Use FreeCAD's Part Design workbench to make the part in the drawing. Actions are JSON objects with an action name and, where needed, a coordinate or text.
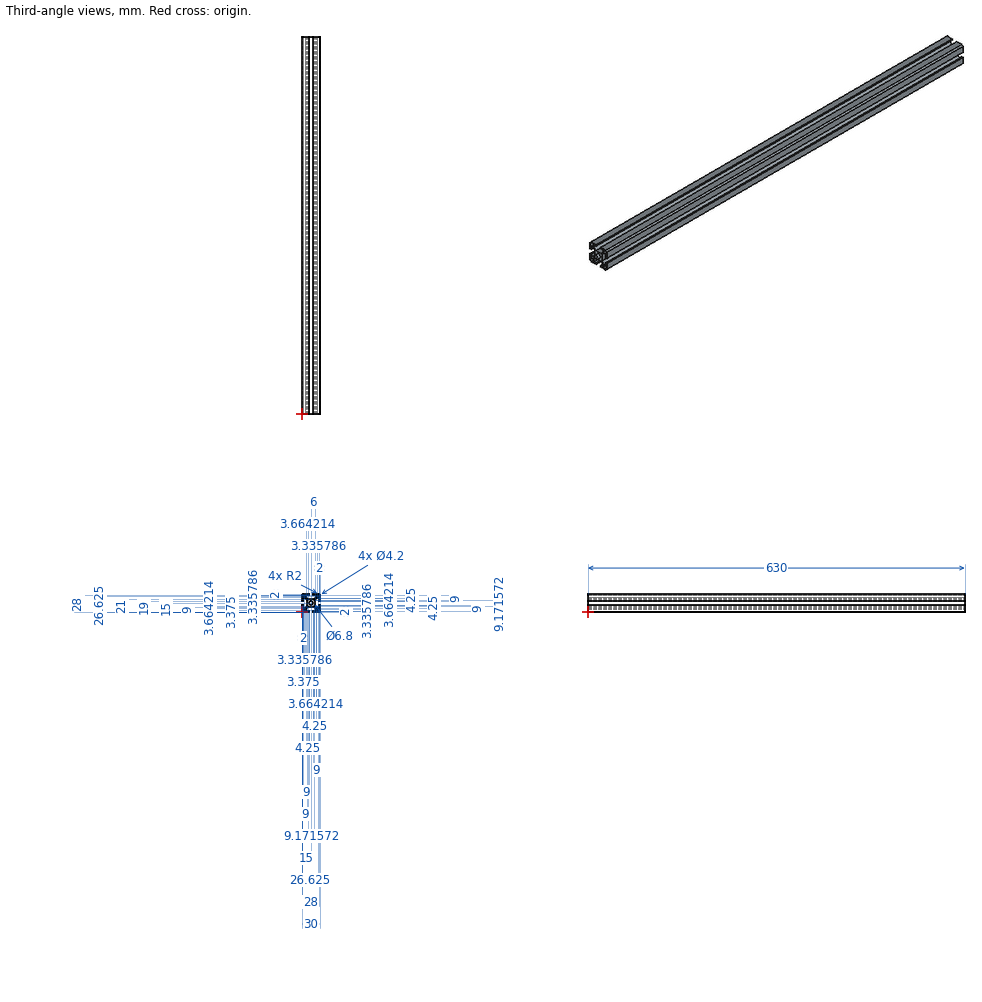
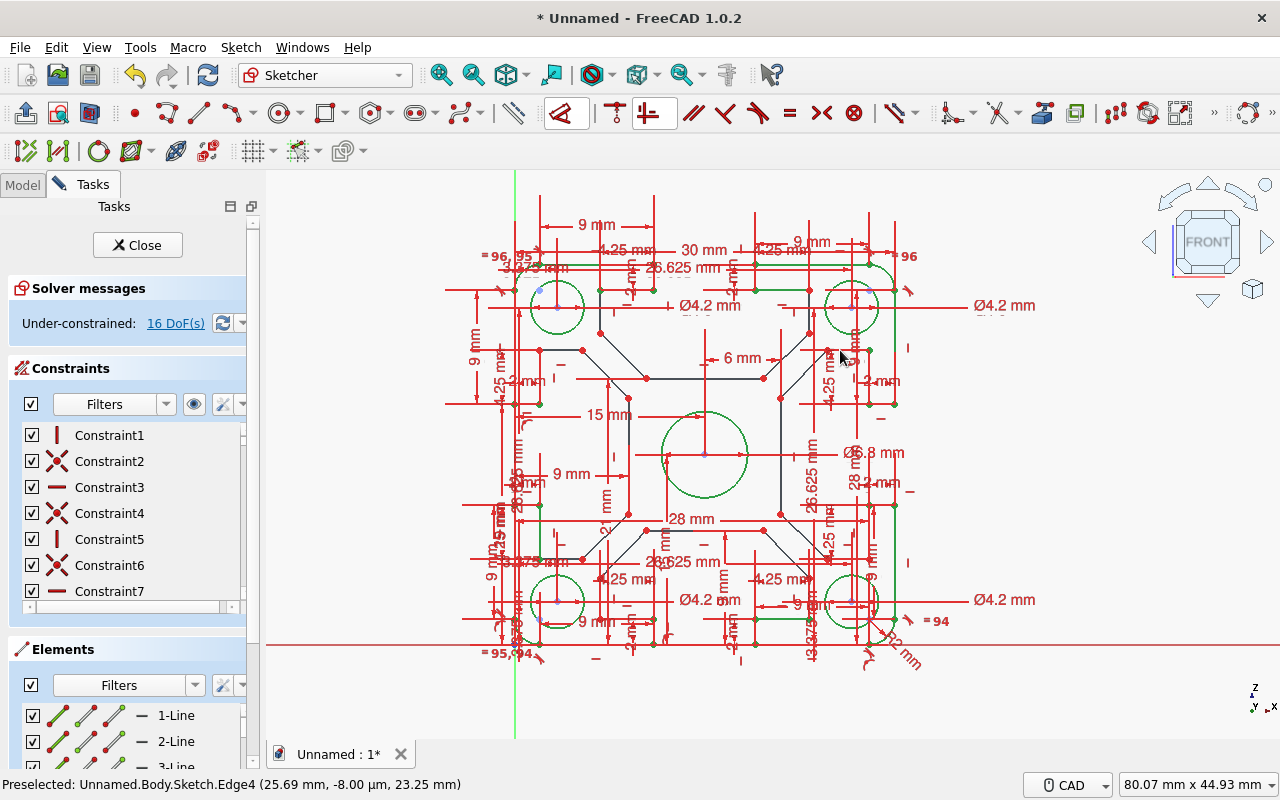
{"action": "left_click", "coordinate": [584, 114]}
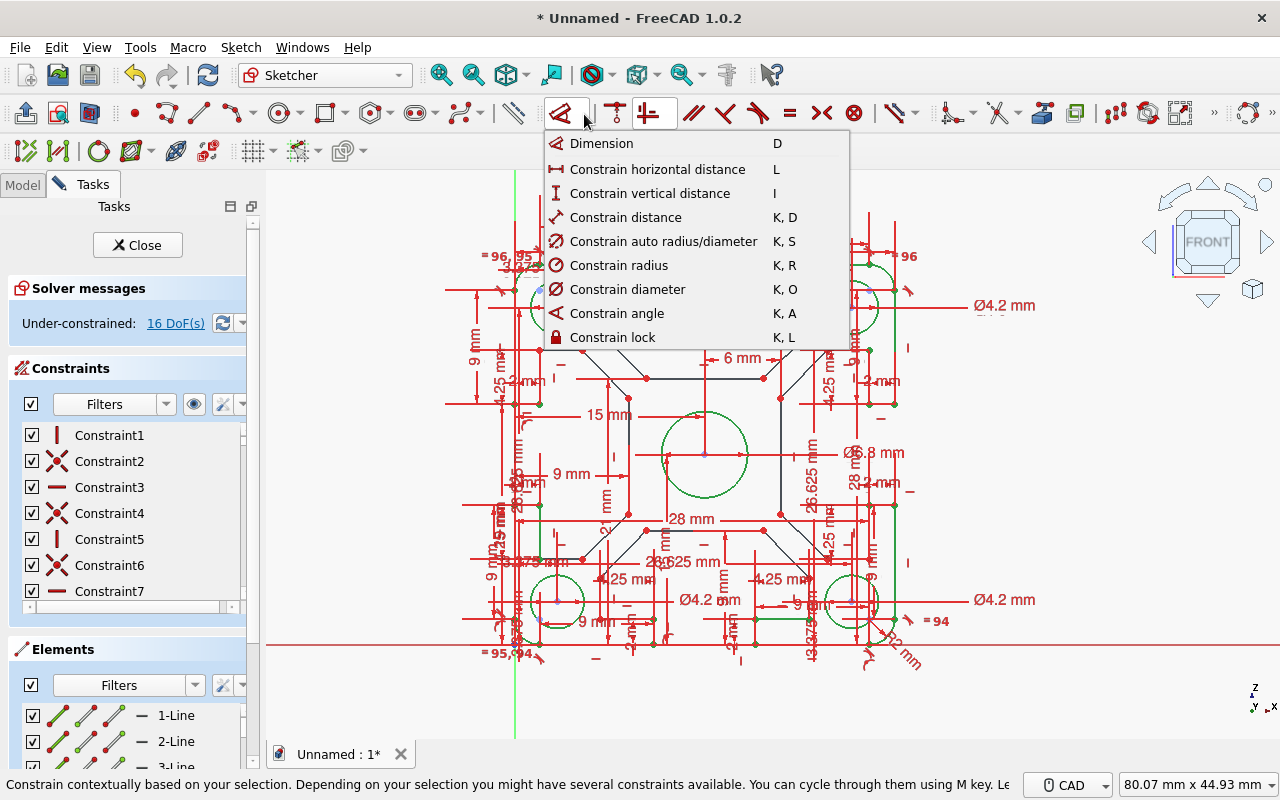
{"action": "left_click", "coordinate": [697, 169]}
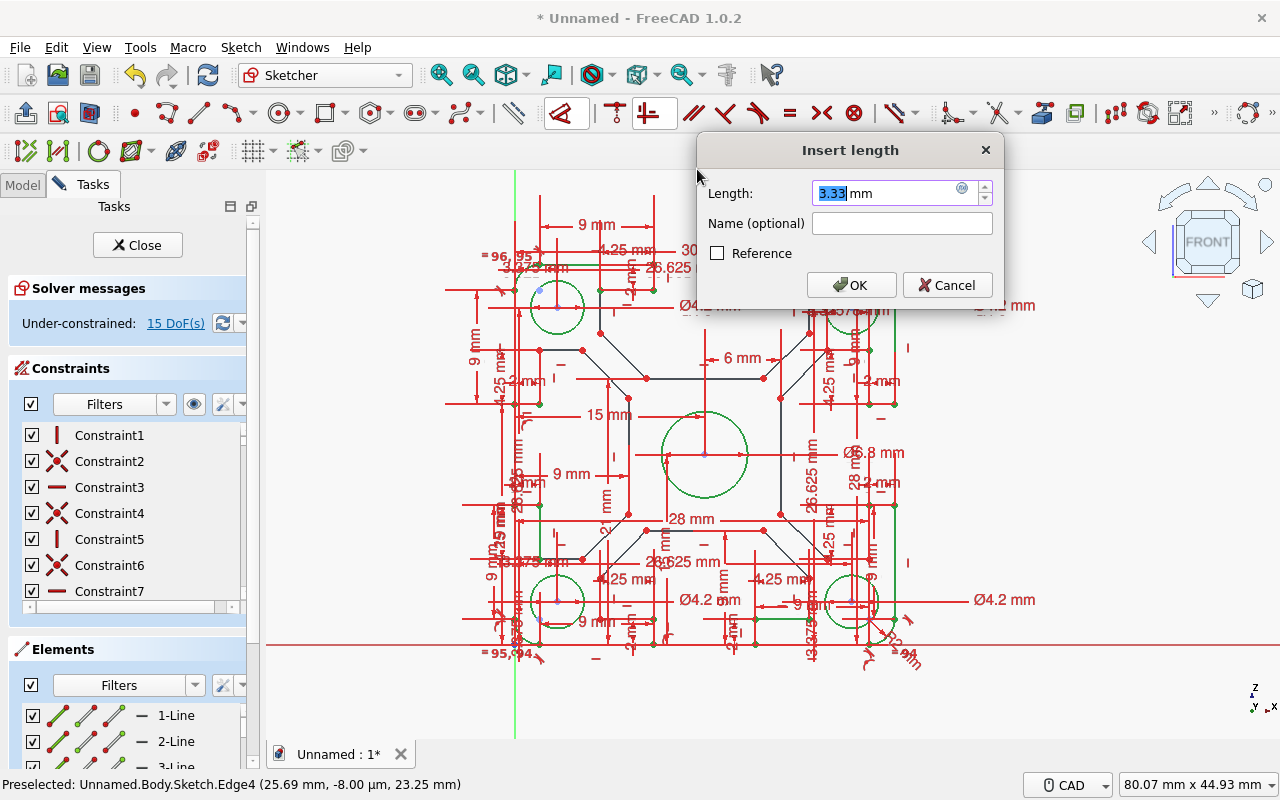
{"action": "type", "text": "3.335786"}
{"action": "key", "text": "Return"}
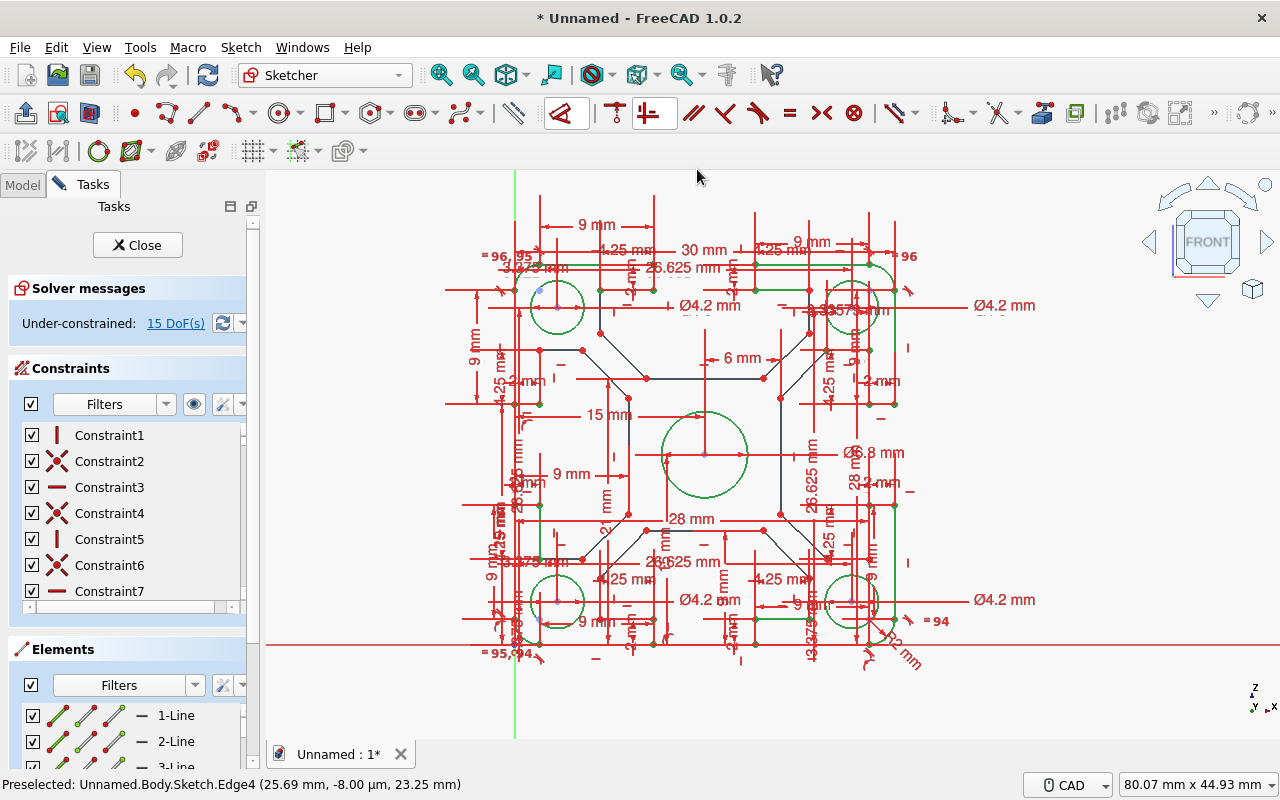
{"action": "left_click", "coordinate": [781, 433]}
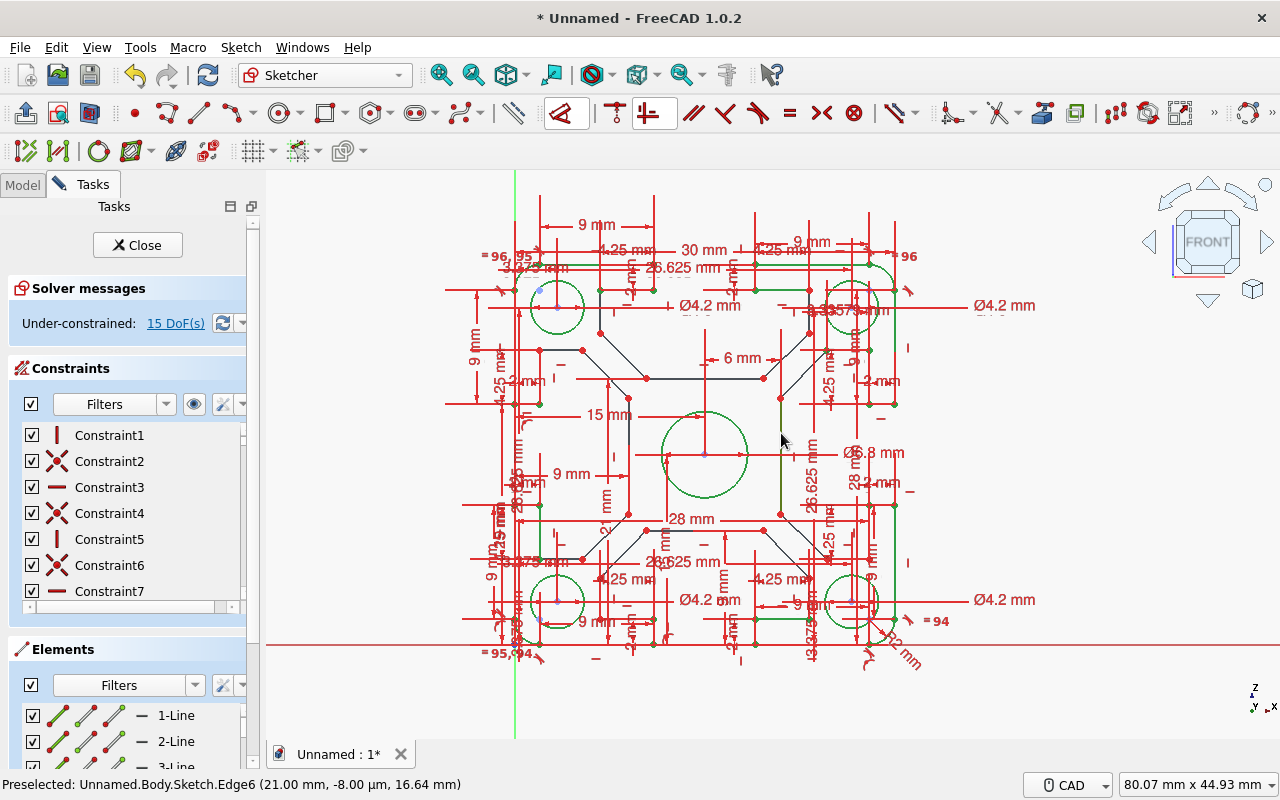
{"action": "key", "text": "i"}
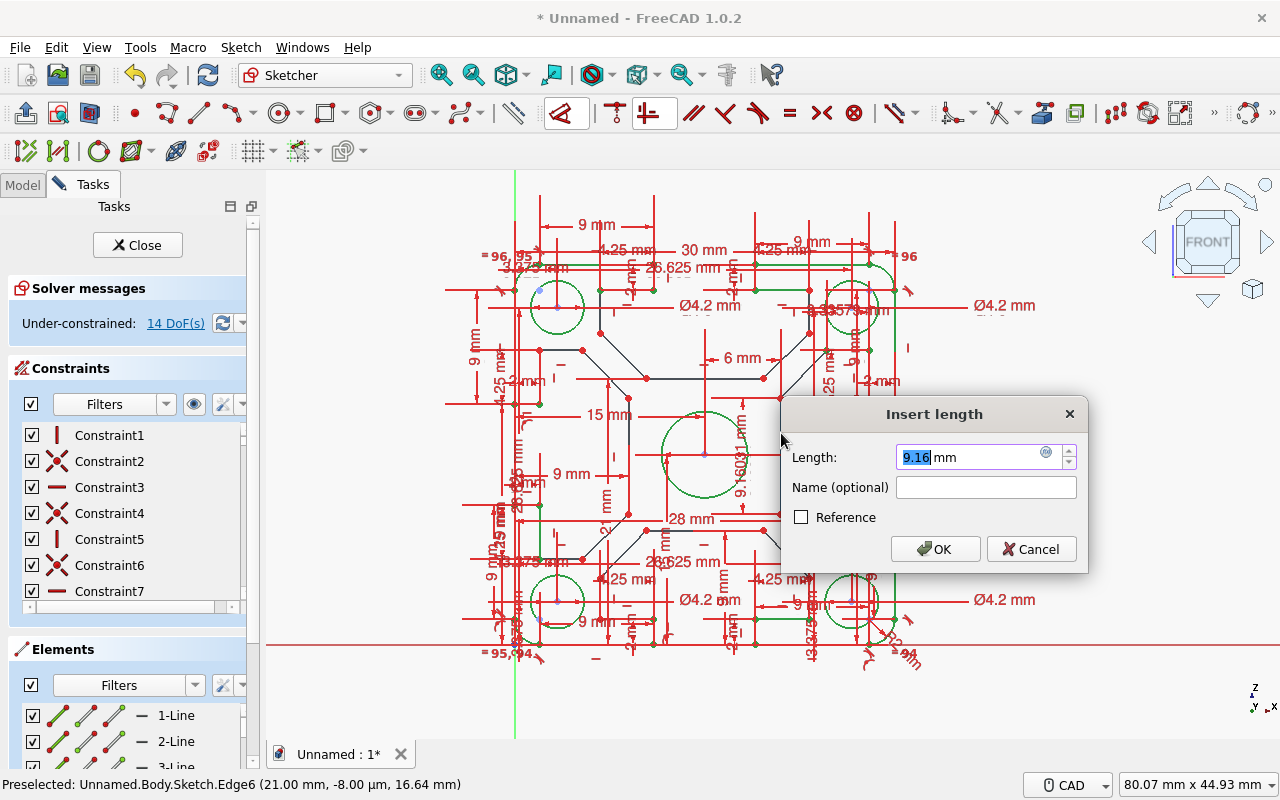
{"action": "type", "text": "9.171572"}
{"action": "key", "text": "Return"}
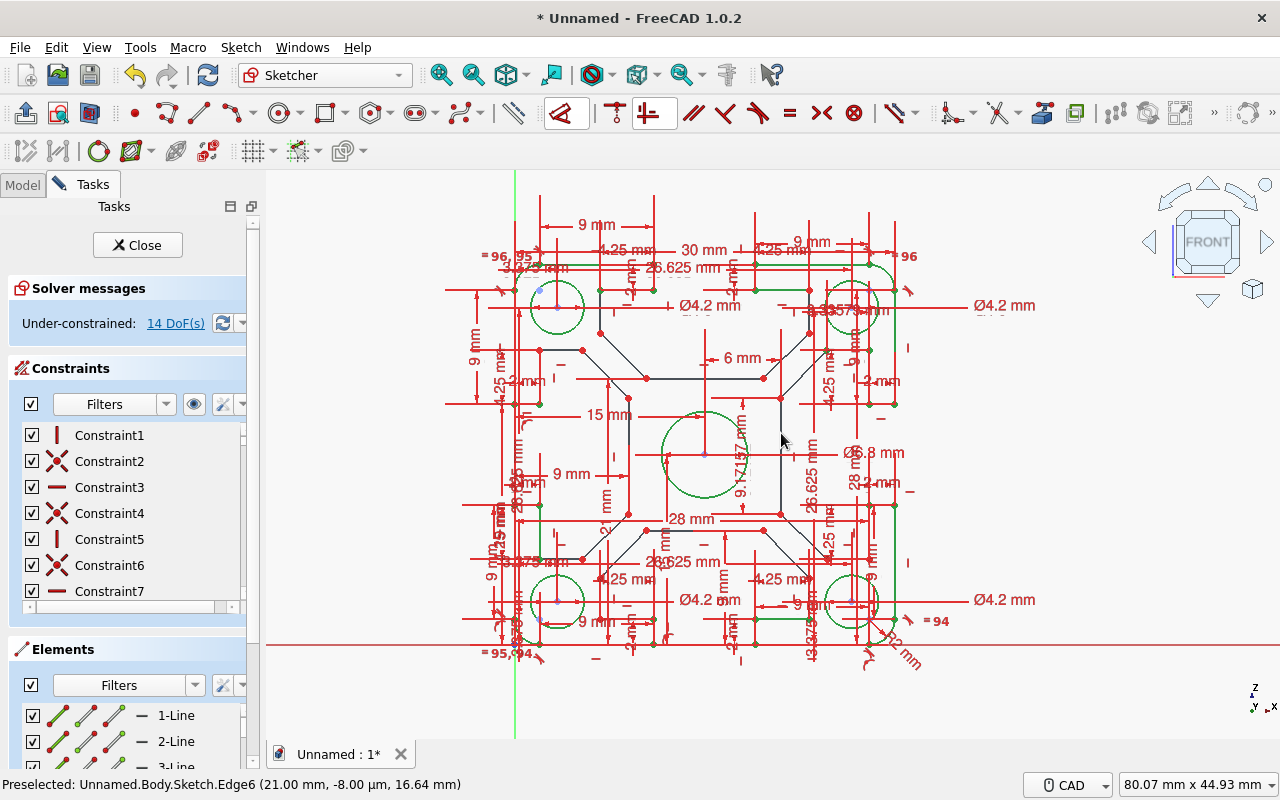
{"action": "left_click", "coordinate": [840, 559]}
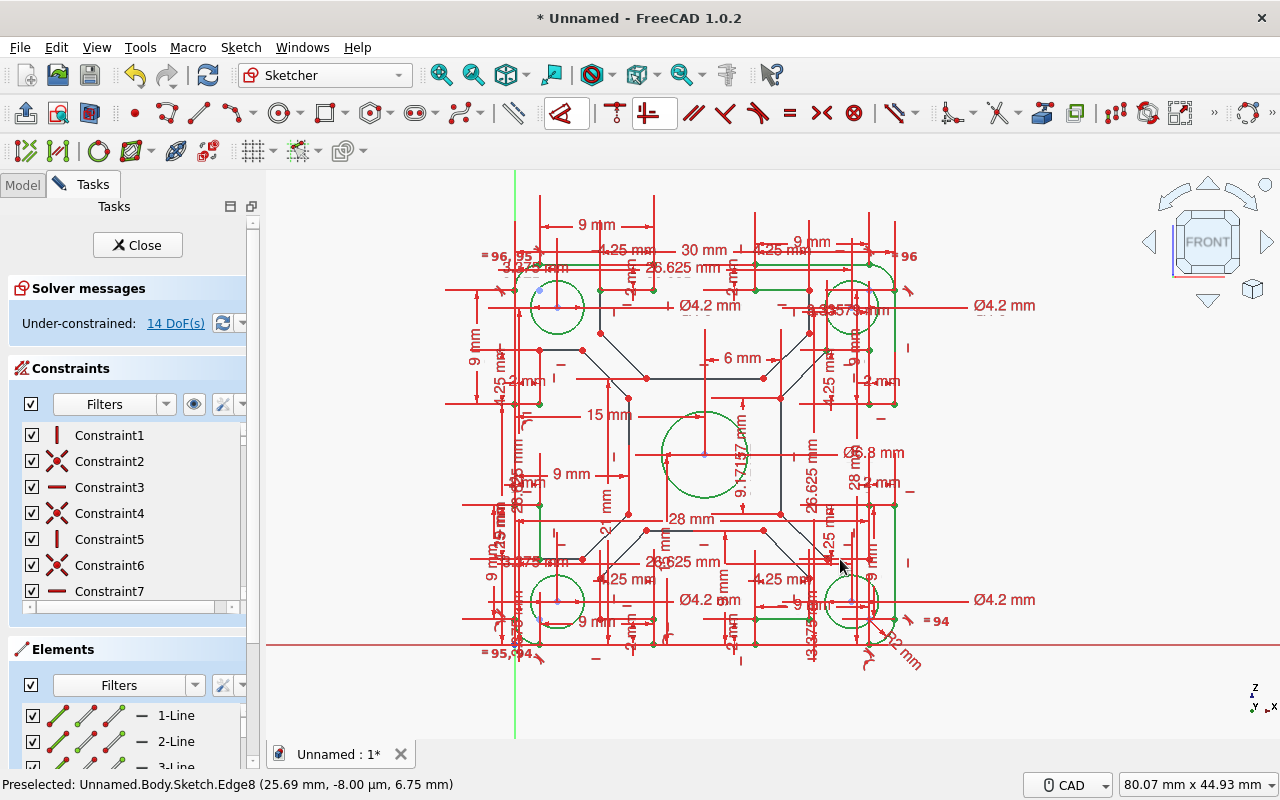
{"action": "key", "text": "l"}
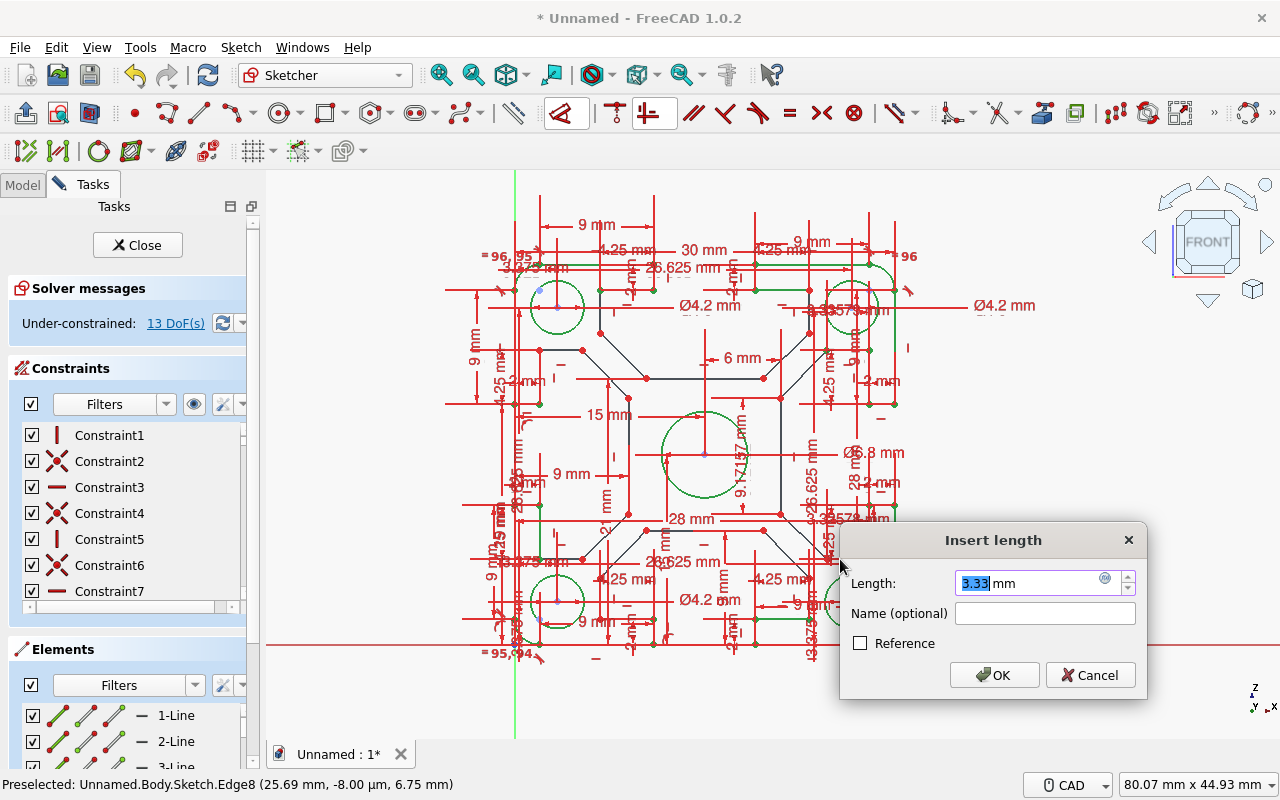
{"action": "type", "text": "3.335786"}
{"action": "key", "text": "Return"}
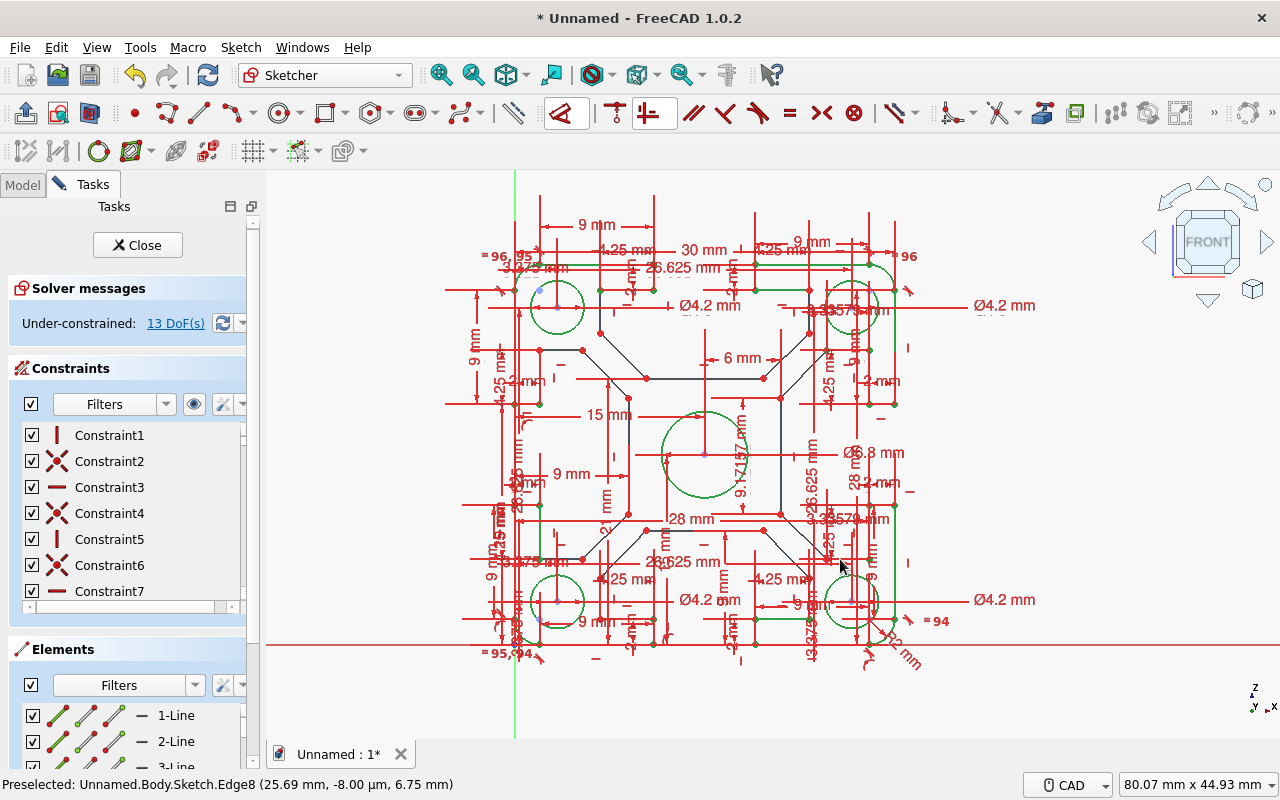
{"action": "scroll", "coordinate": [809, 607], "scroll_direction": "up", "scroll_amount": 4}